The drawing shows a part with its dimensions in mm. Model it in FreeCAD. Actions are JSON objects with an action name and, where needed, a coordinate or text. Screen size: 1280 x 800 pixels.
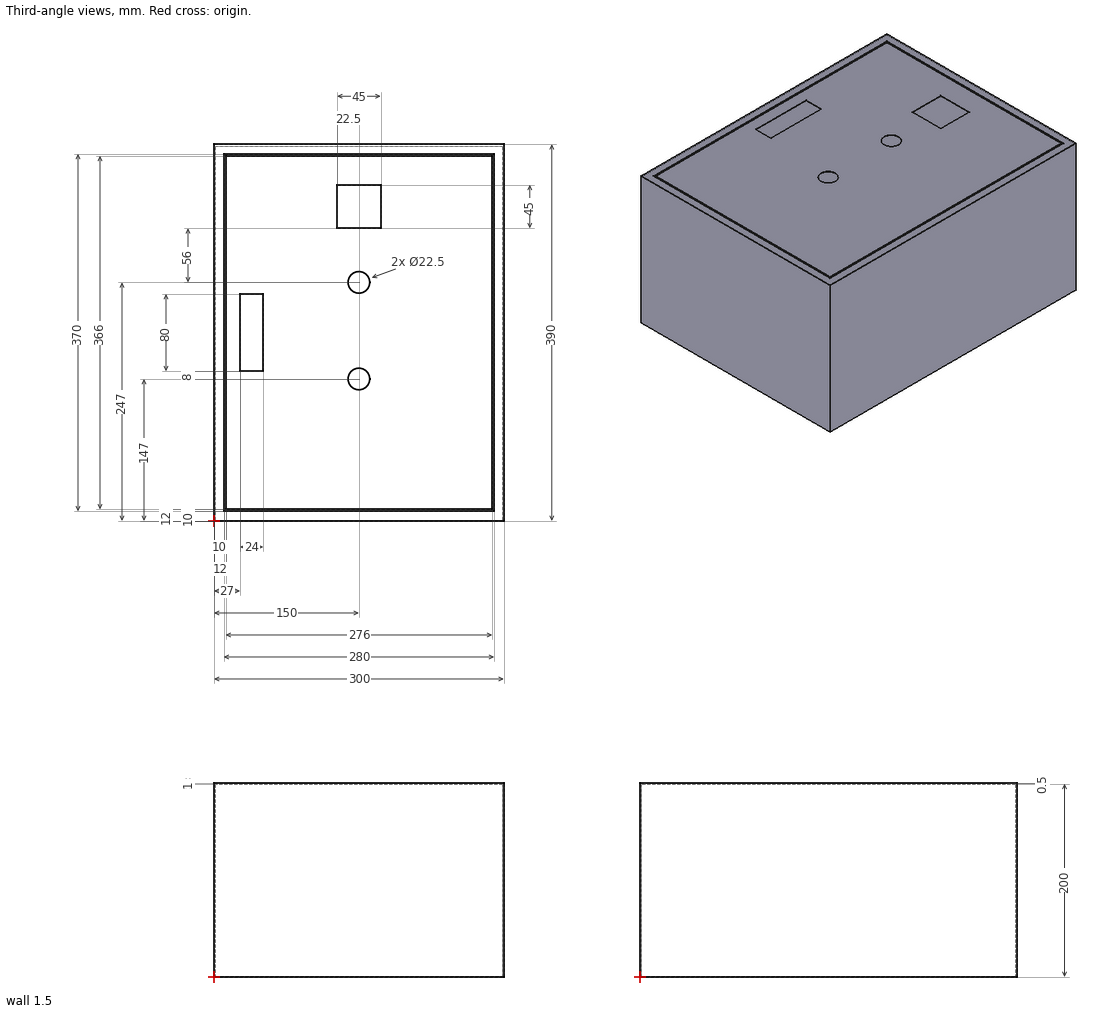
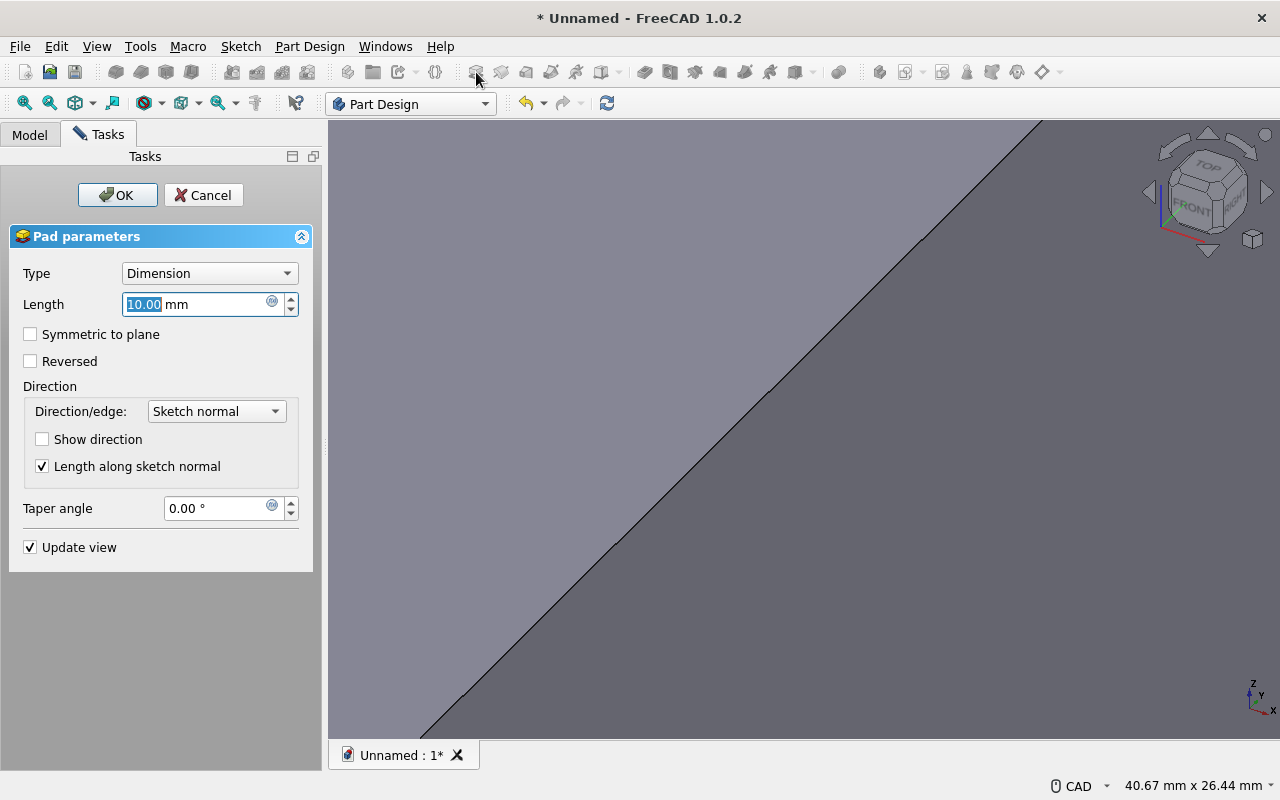
{"action": "type", "text": "1"}
{"action": "key", "text": "Tab"}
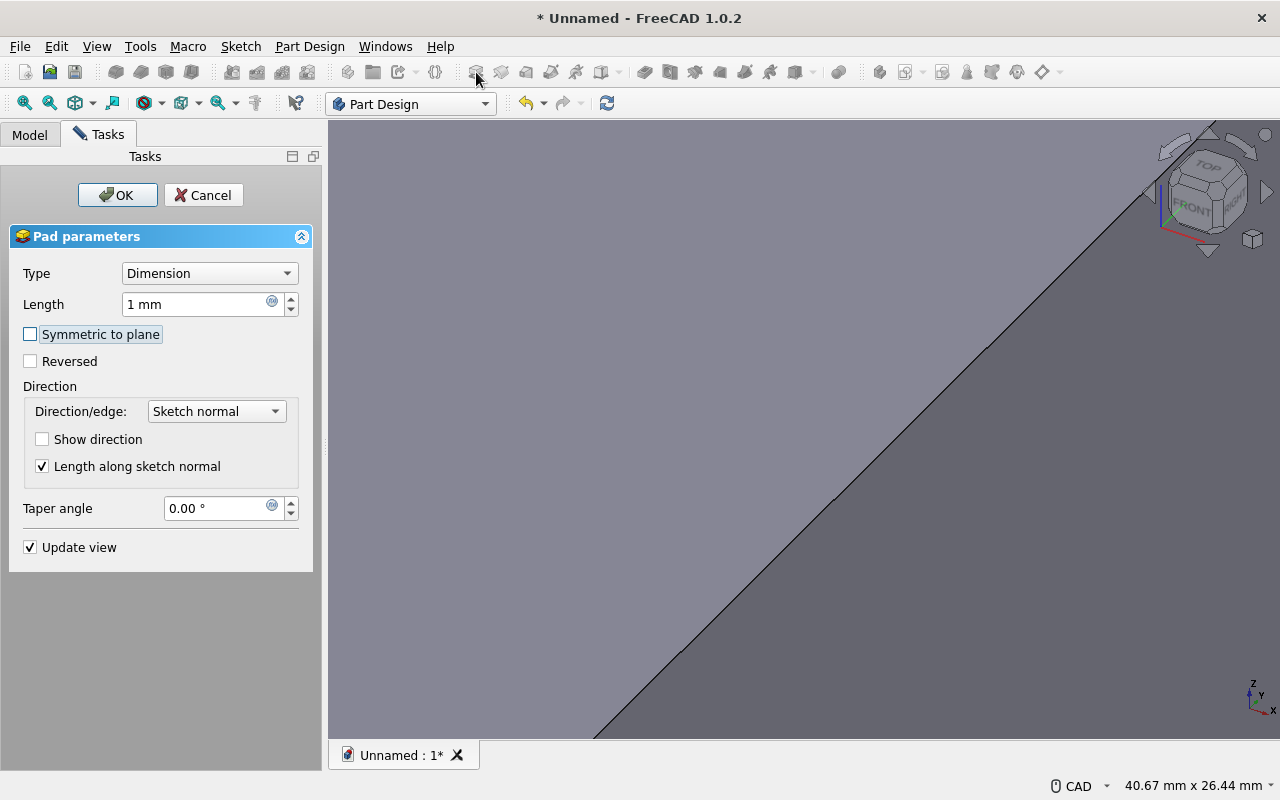
{"action": "left_click", "coordinate": [118, 195]}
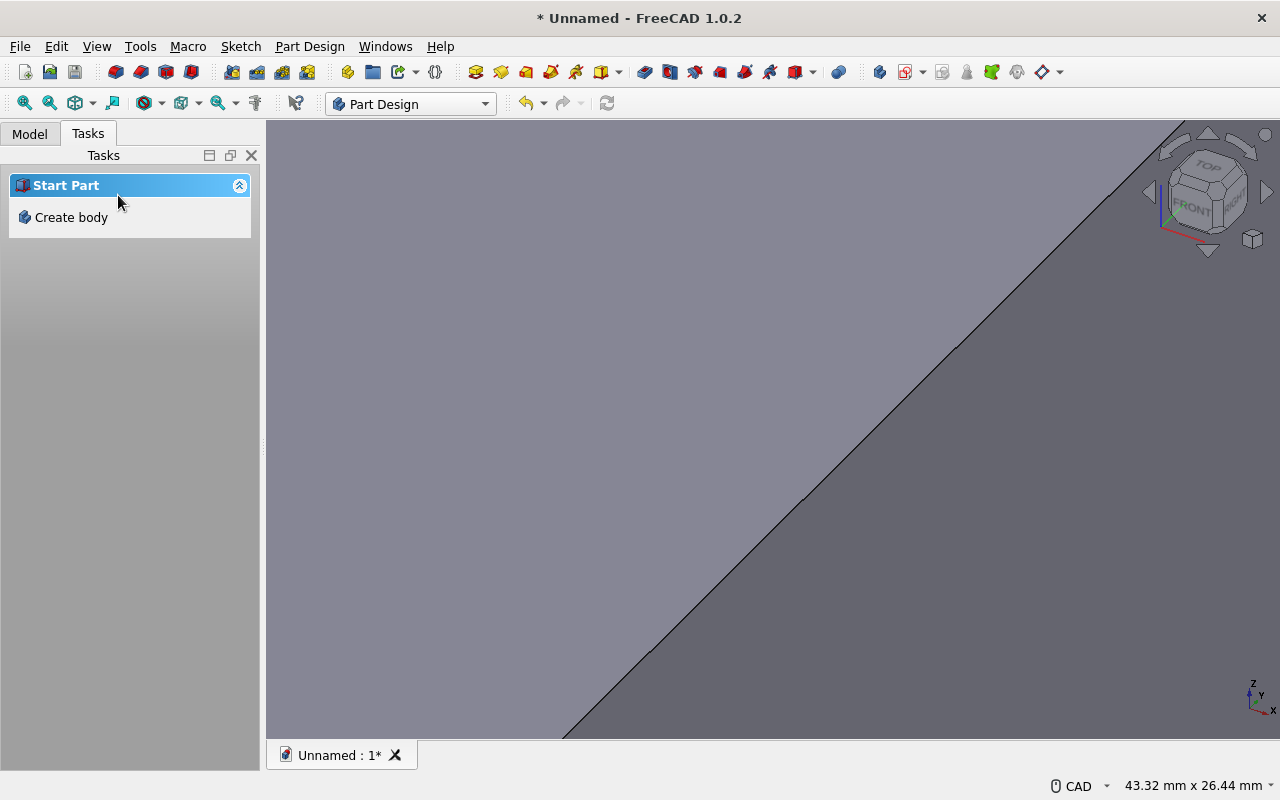
{"action": "left_click", "coordinate": [25, 104]}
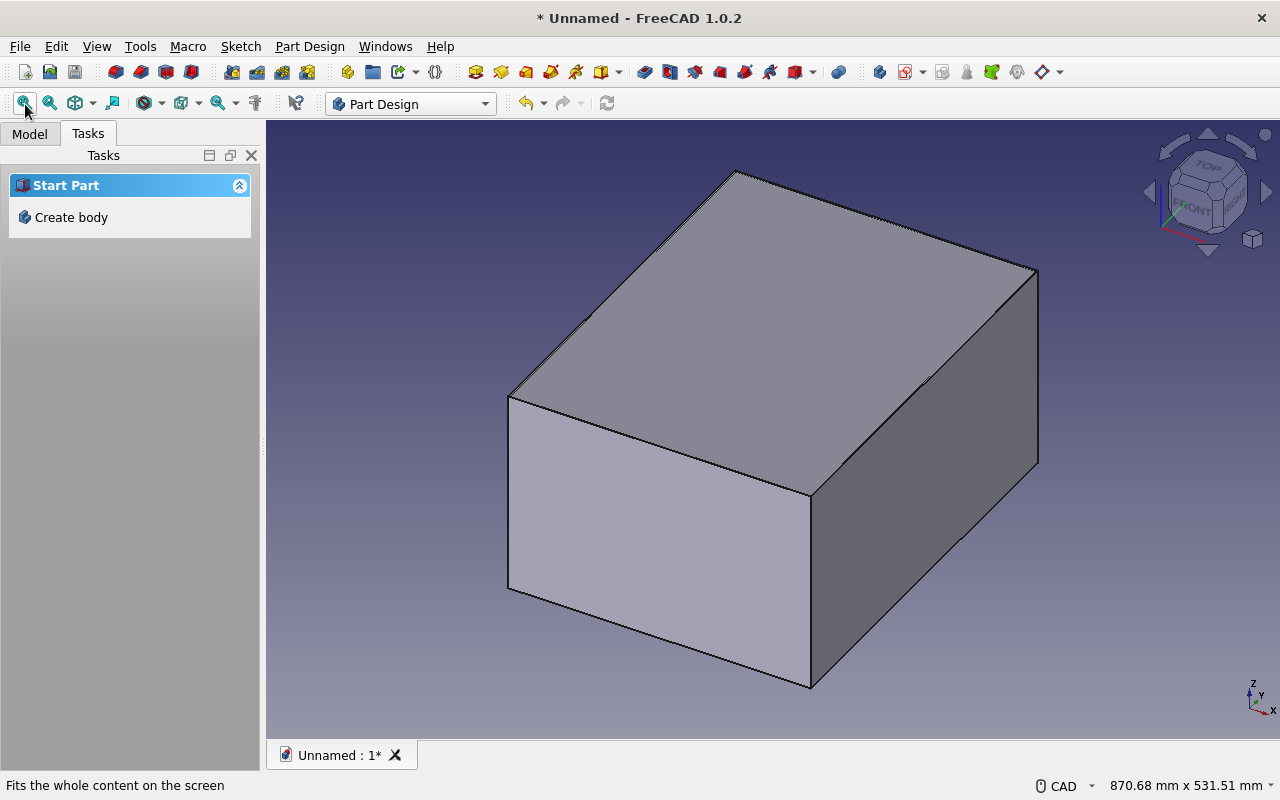
{"action": "left_click", "coordinate": [773, 333]}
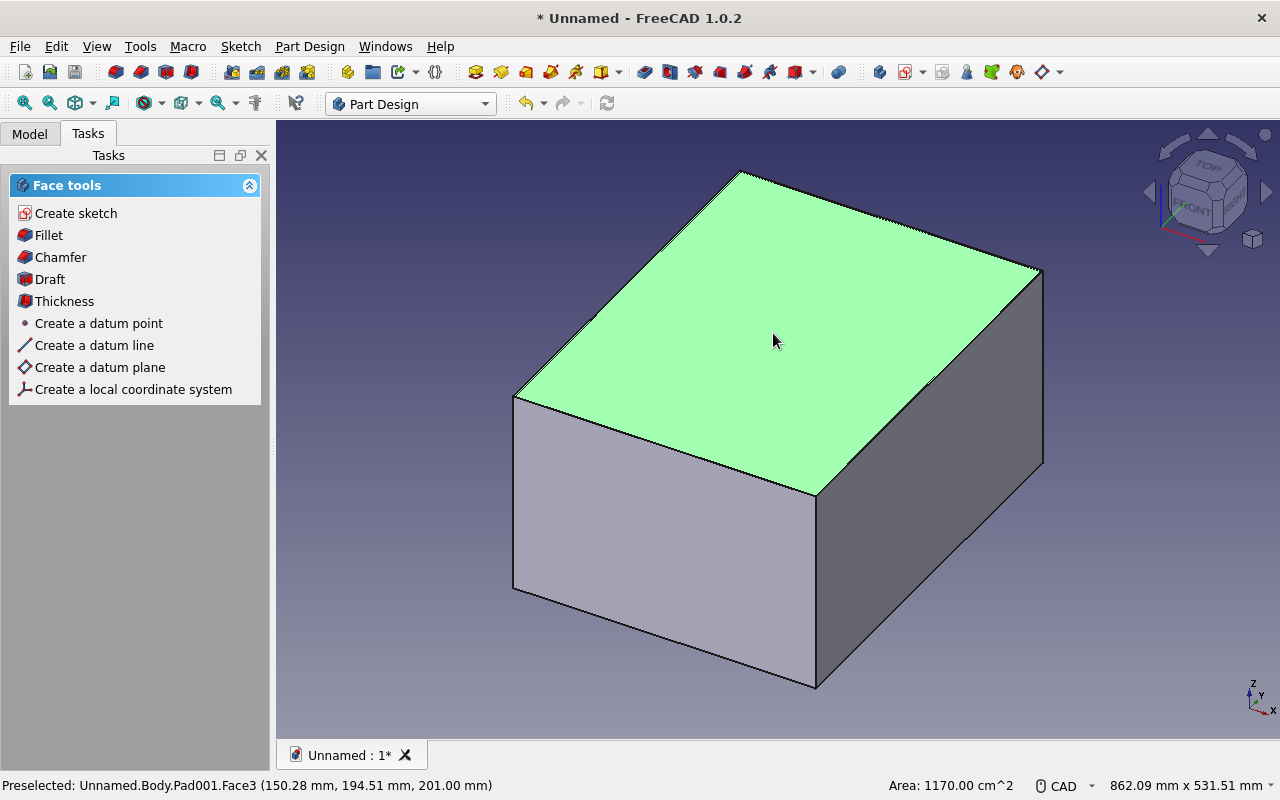
{"action": "left_click", "coordinate": [904, 72]}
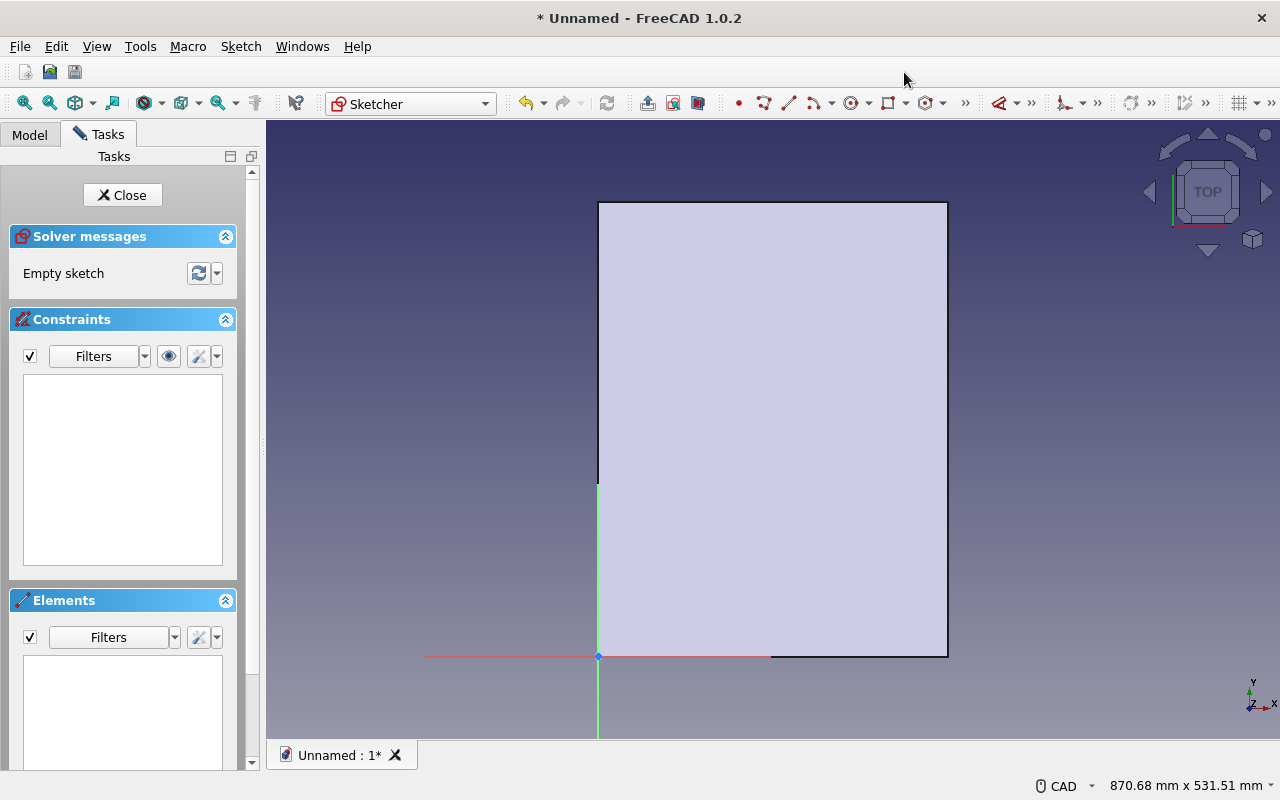
{"action": "left_click", "coordinate": [888, 104]}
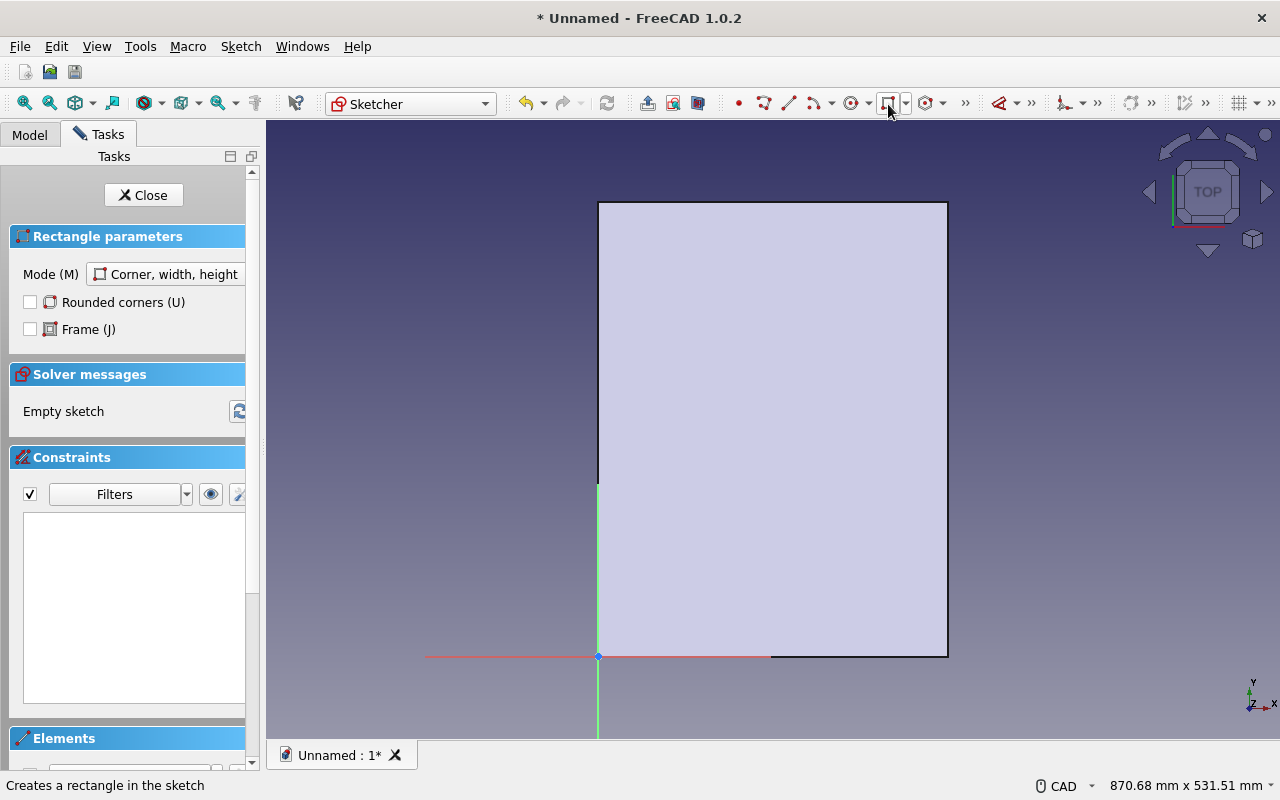
{"action": "scroll", "coordinate": [610, 214], "scroll_direction": "up", "scroll_amount": 2}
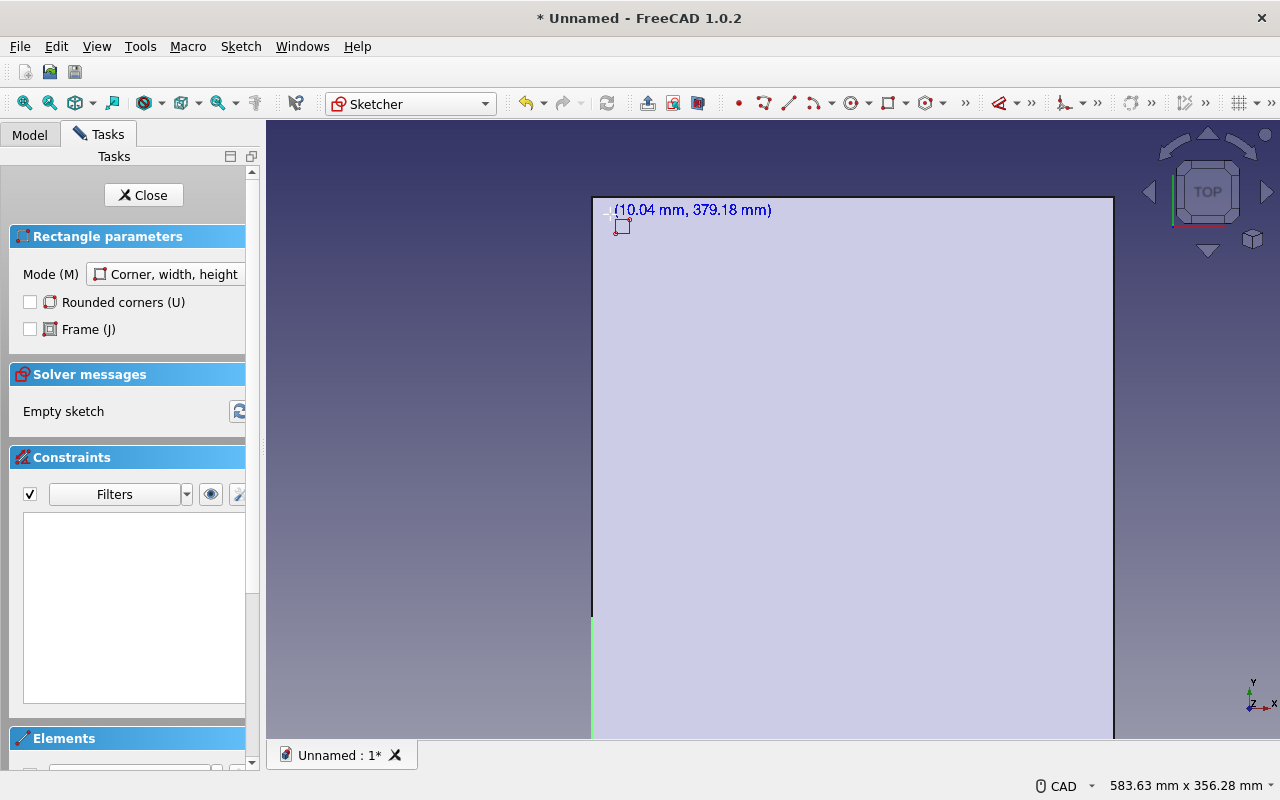
{"action": "left_click", "coordinate": [610, 214]}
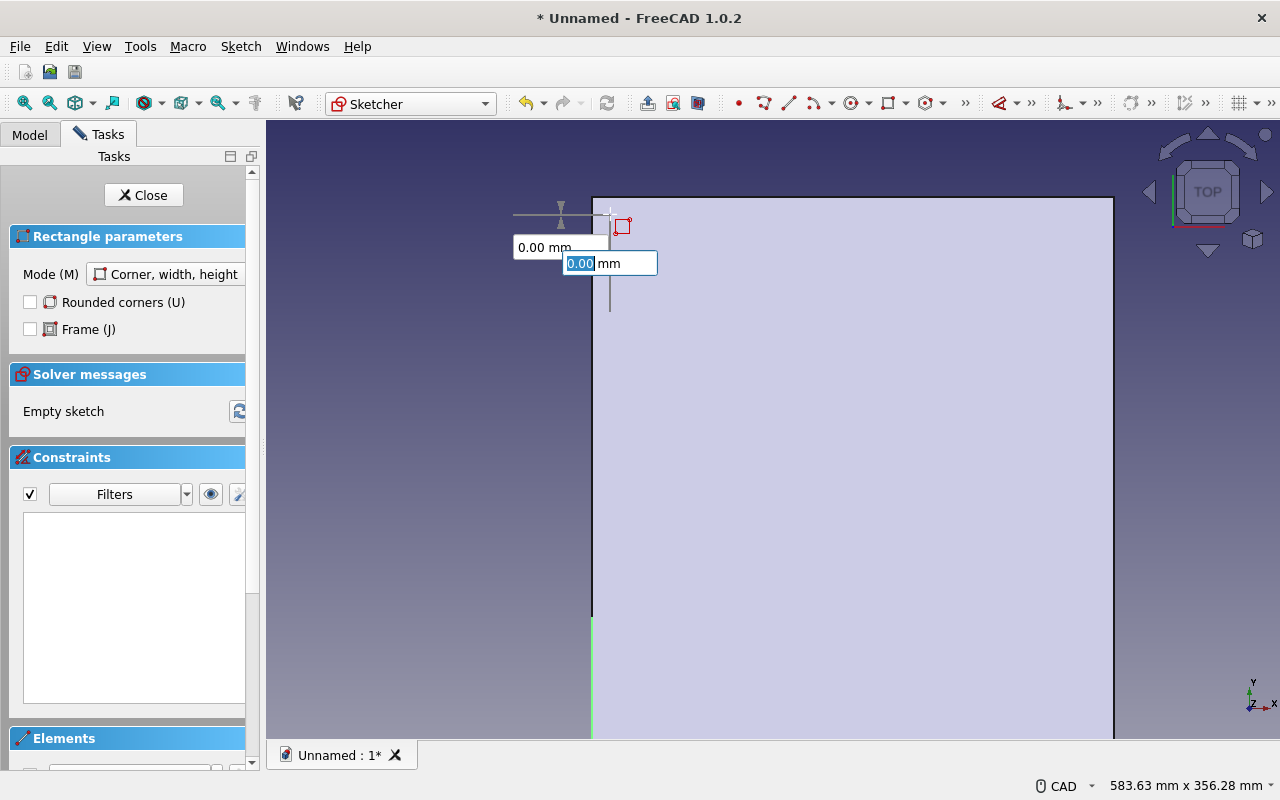
{"action": "scroll", "coordinate": [534, 290], "scroll_direction": "down", "scroll_amount": 3}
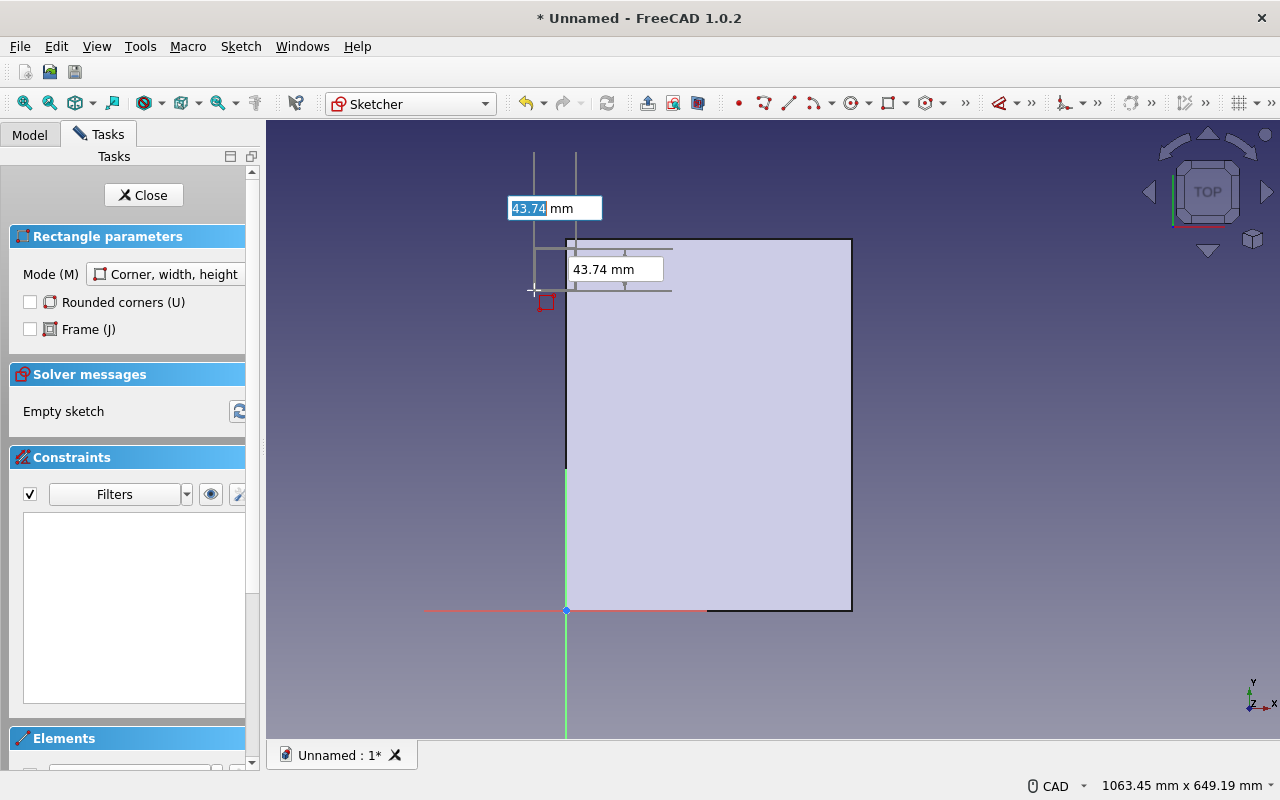
{"action": "scroll", "coordinate": [843, 601], "scroll_direction": "up", "scroll_amount": 3}